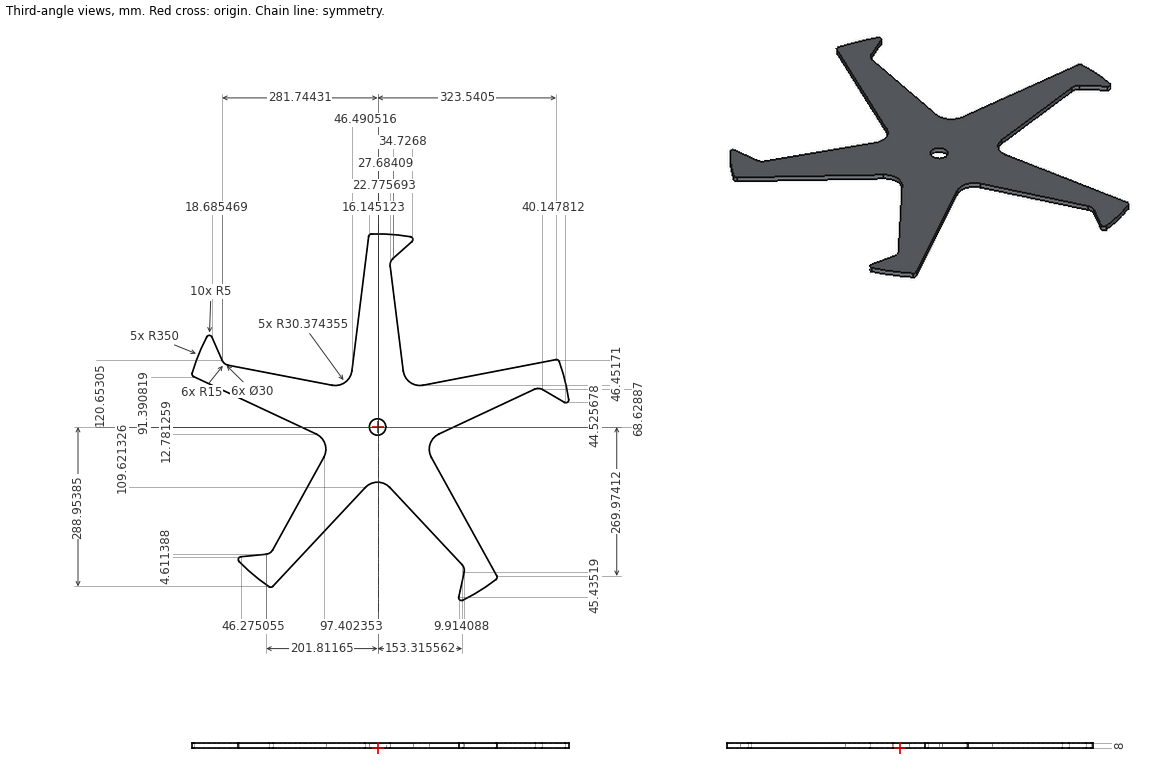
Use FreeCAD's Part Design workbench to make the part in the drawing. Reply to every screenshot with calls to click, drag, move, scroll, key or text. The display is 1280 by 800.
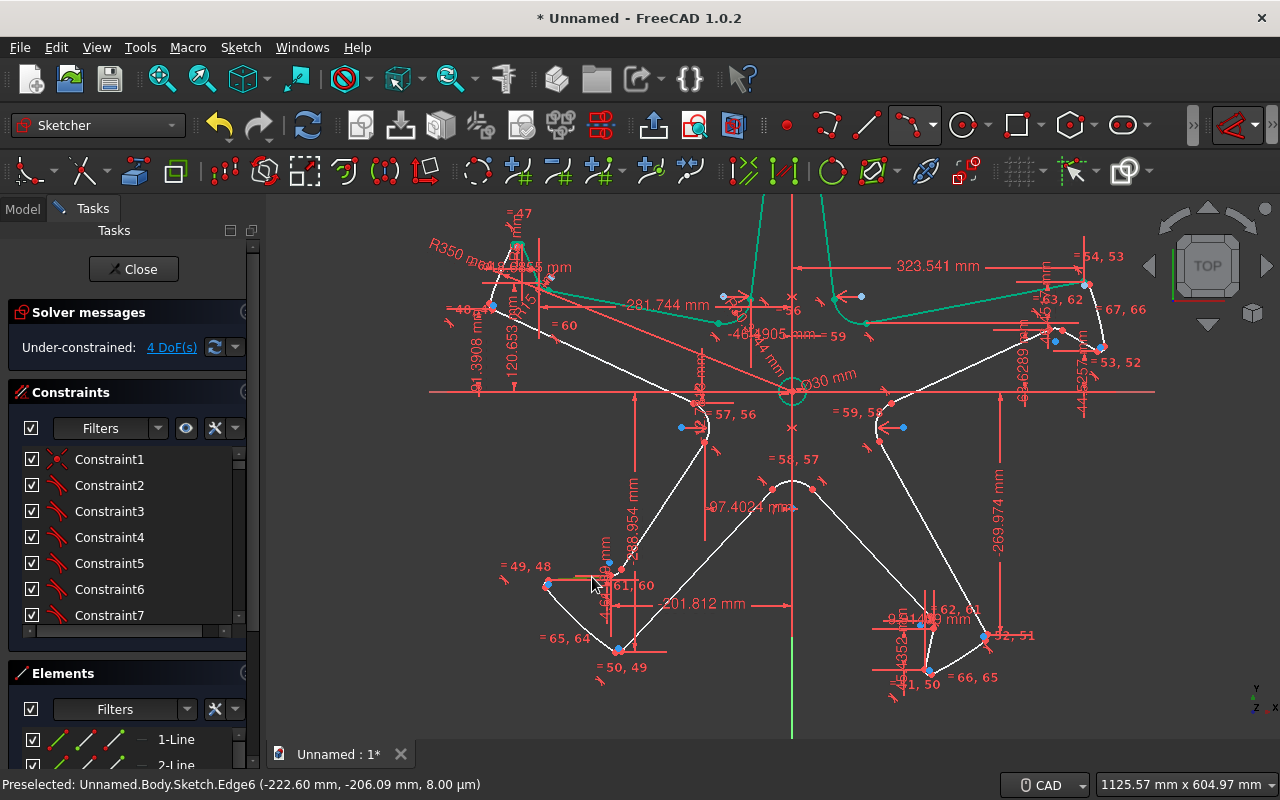
key(l)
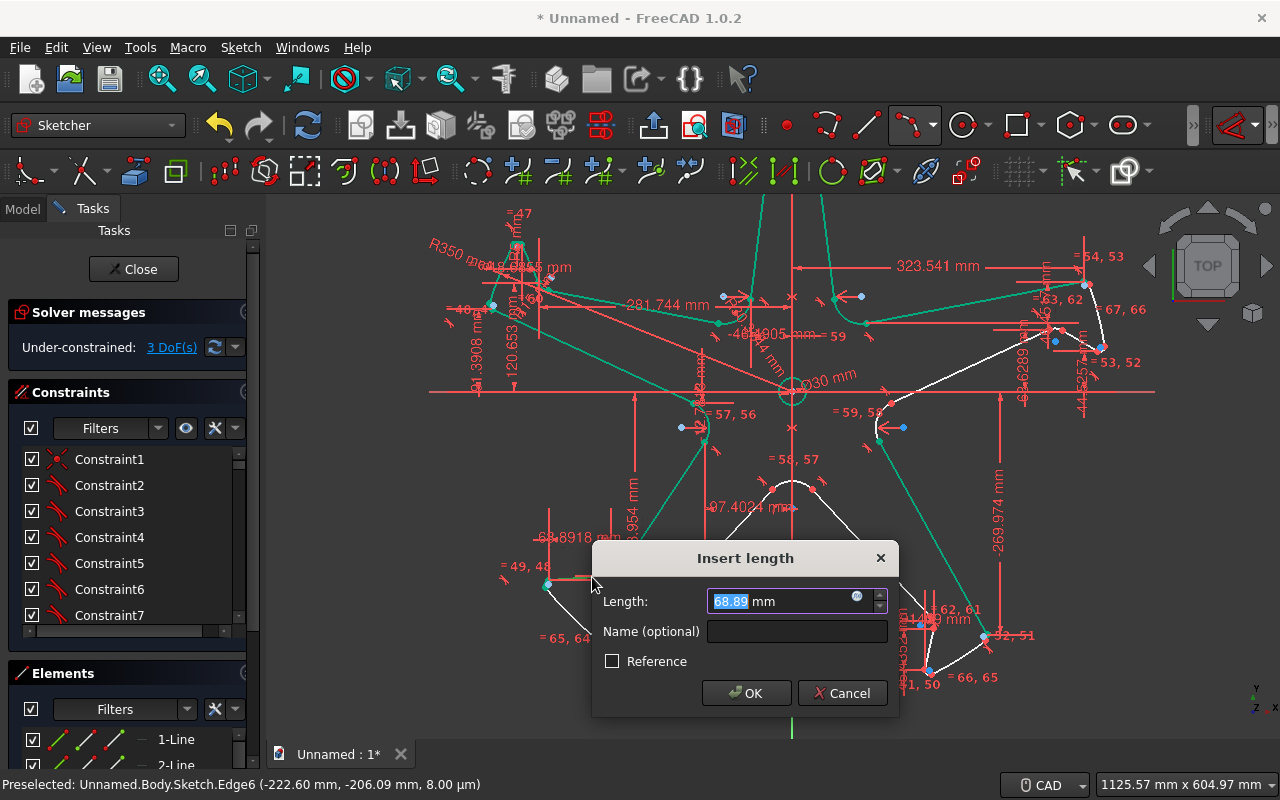
text(46.275055)
key(Return)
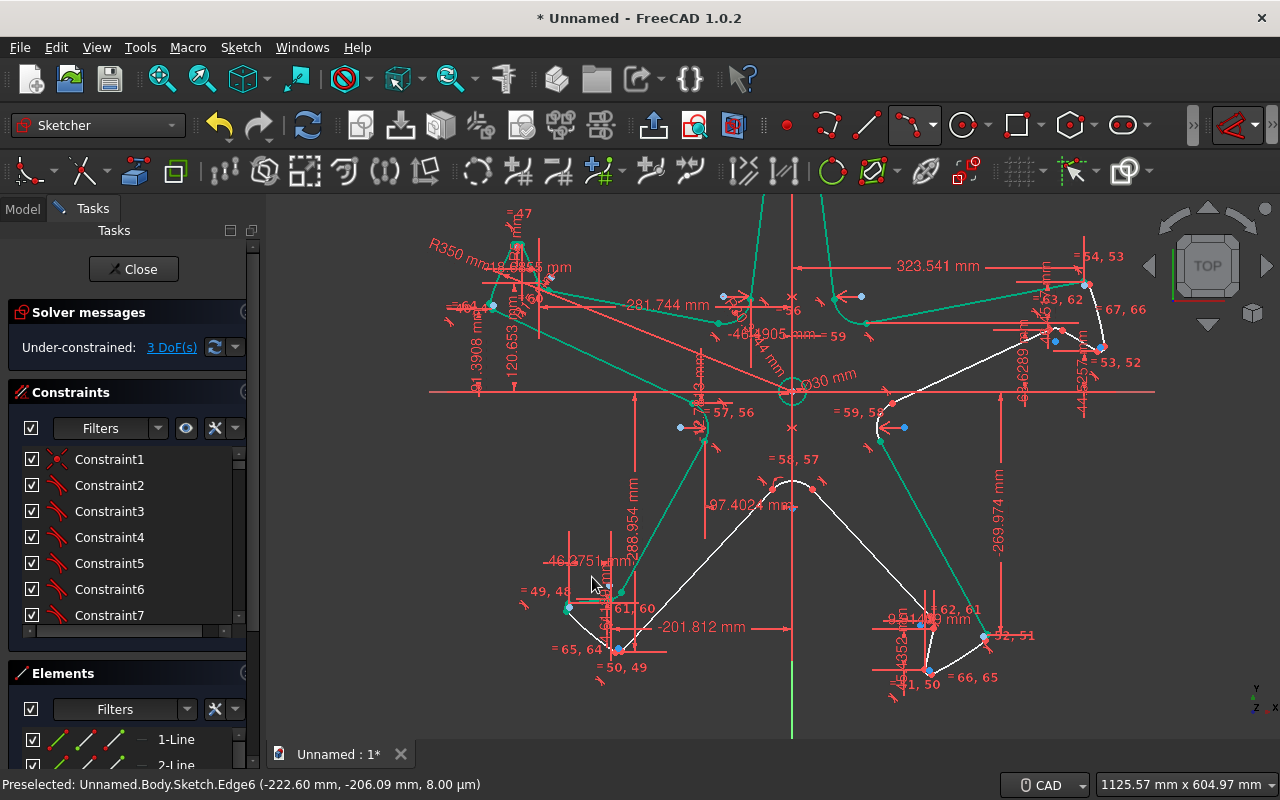
click(1073, 337)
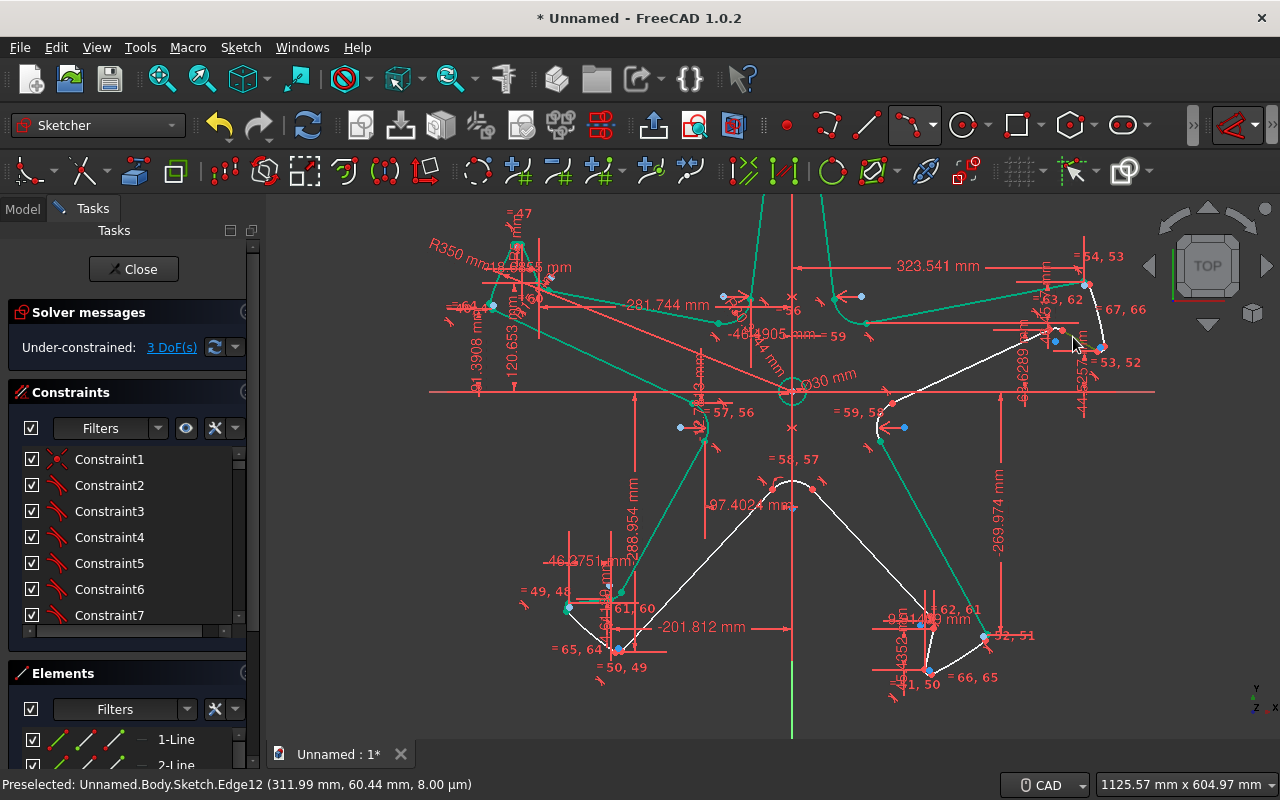
key(l)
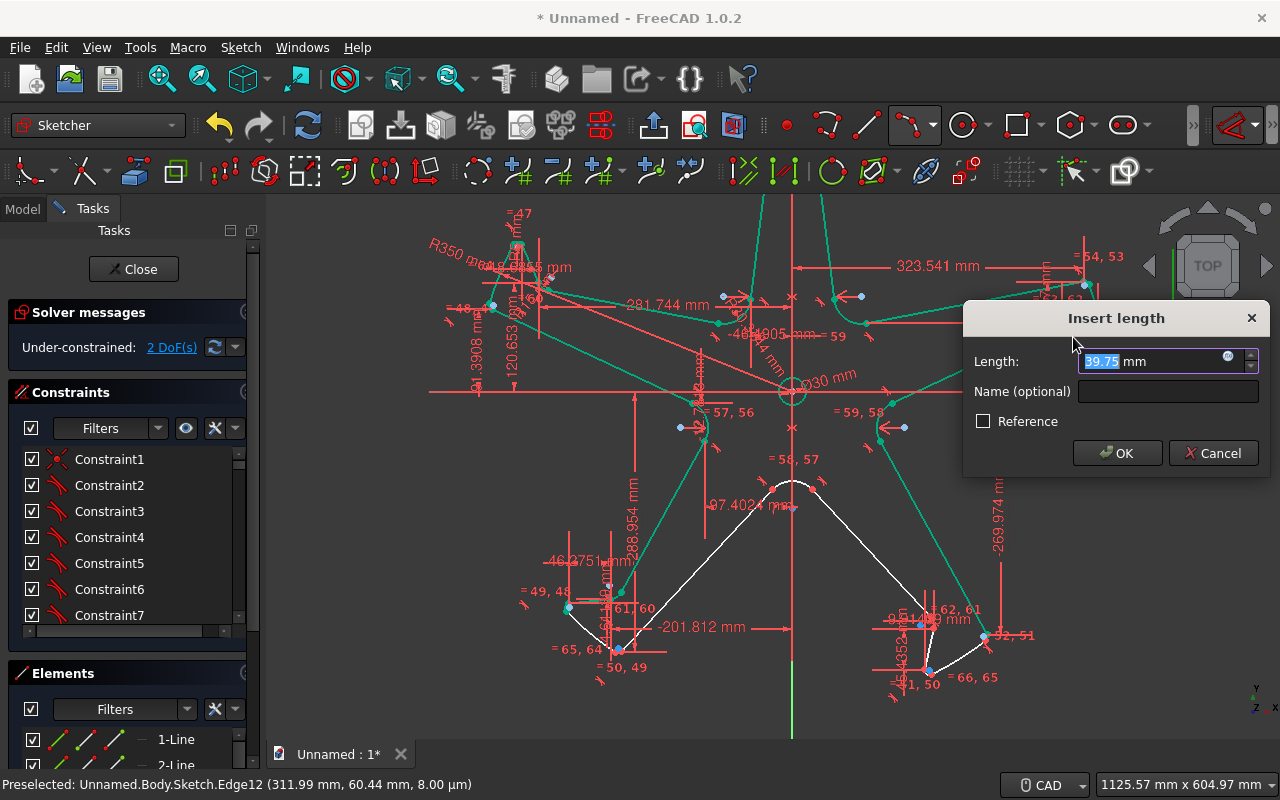
text(40.147812)
key(Return)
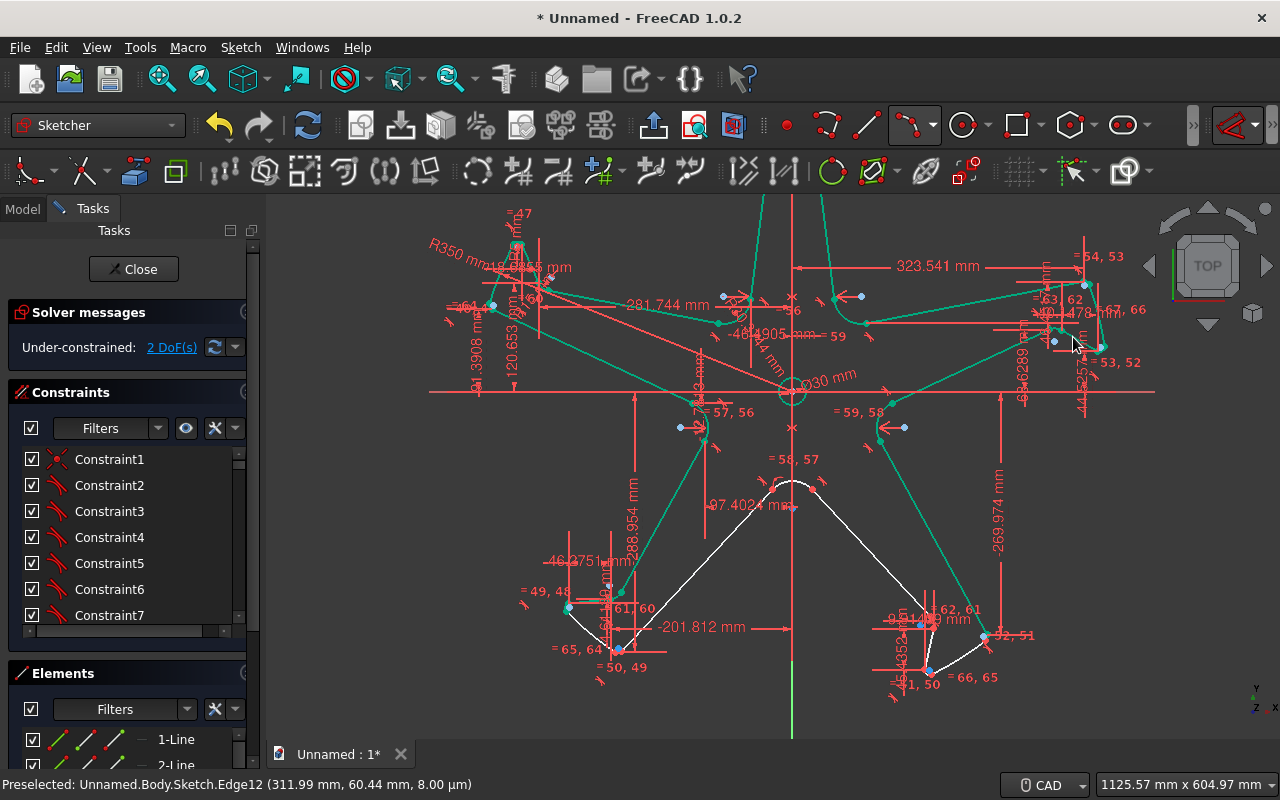
click(772, 490)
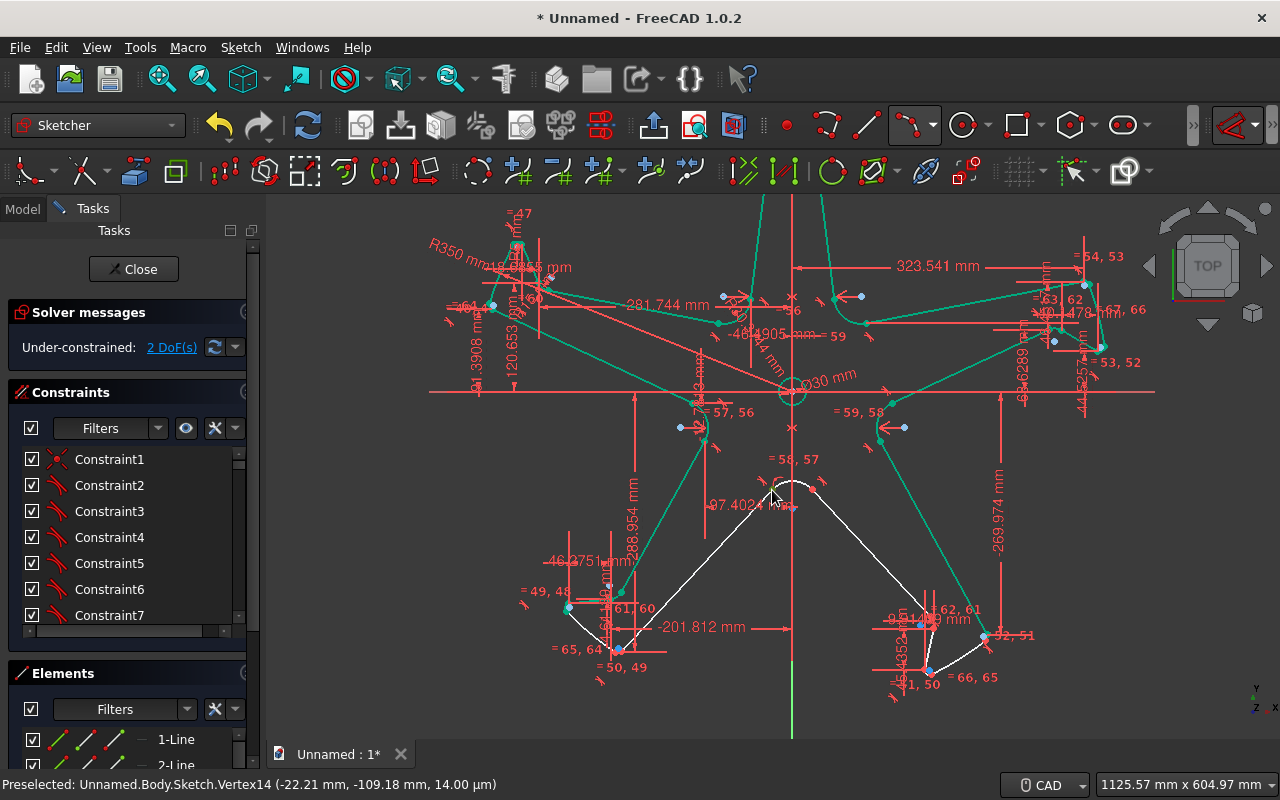
key(i)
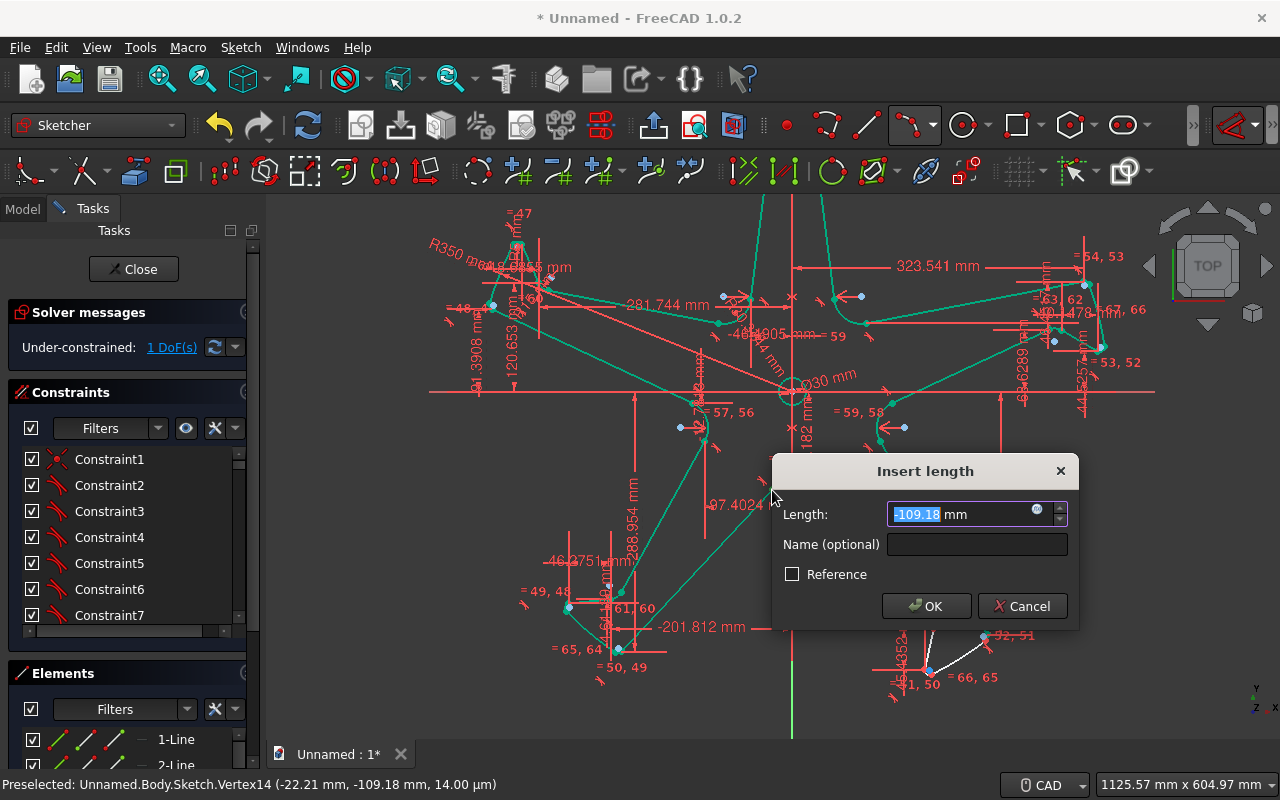
text(-109.621326)
key(Return)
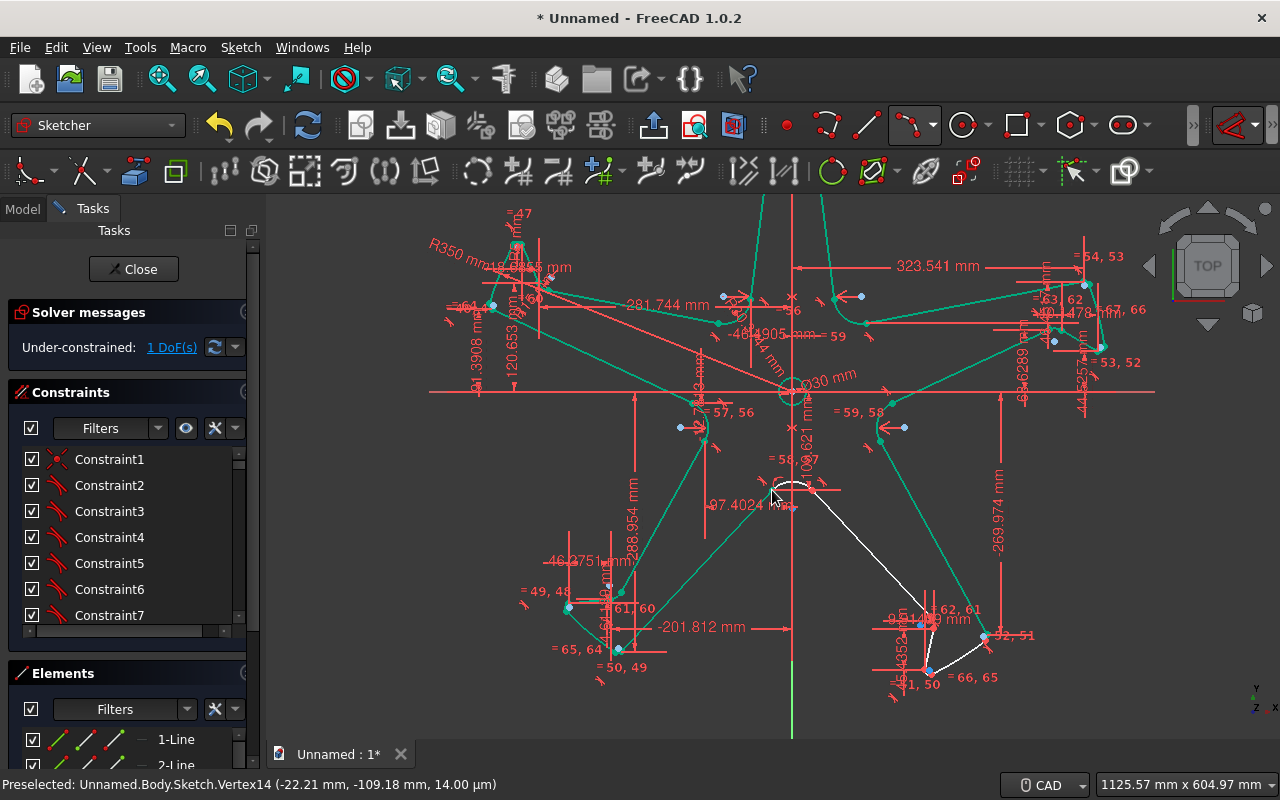
click(930, 617)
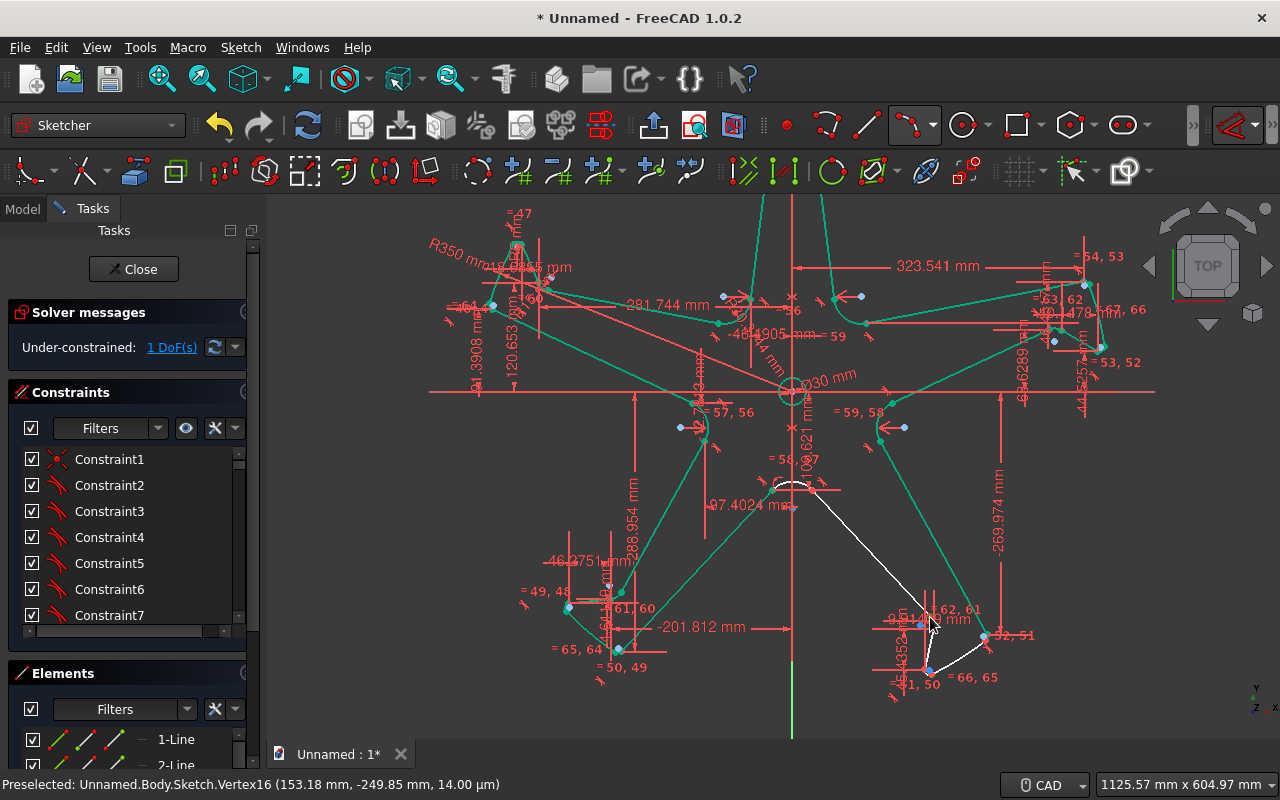
key(l)